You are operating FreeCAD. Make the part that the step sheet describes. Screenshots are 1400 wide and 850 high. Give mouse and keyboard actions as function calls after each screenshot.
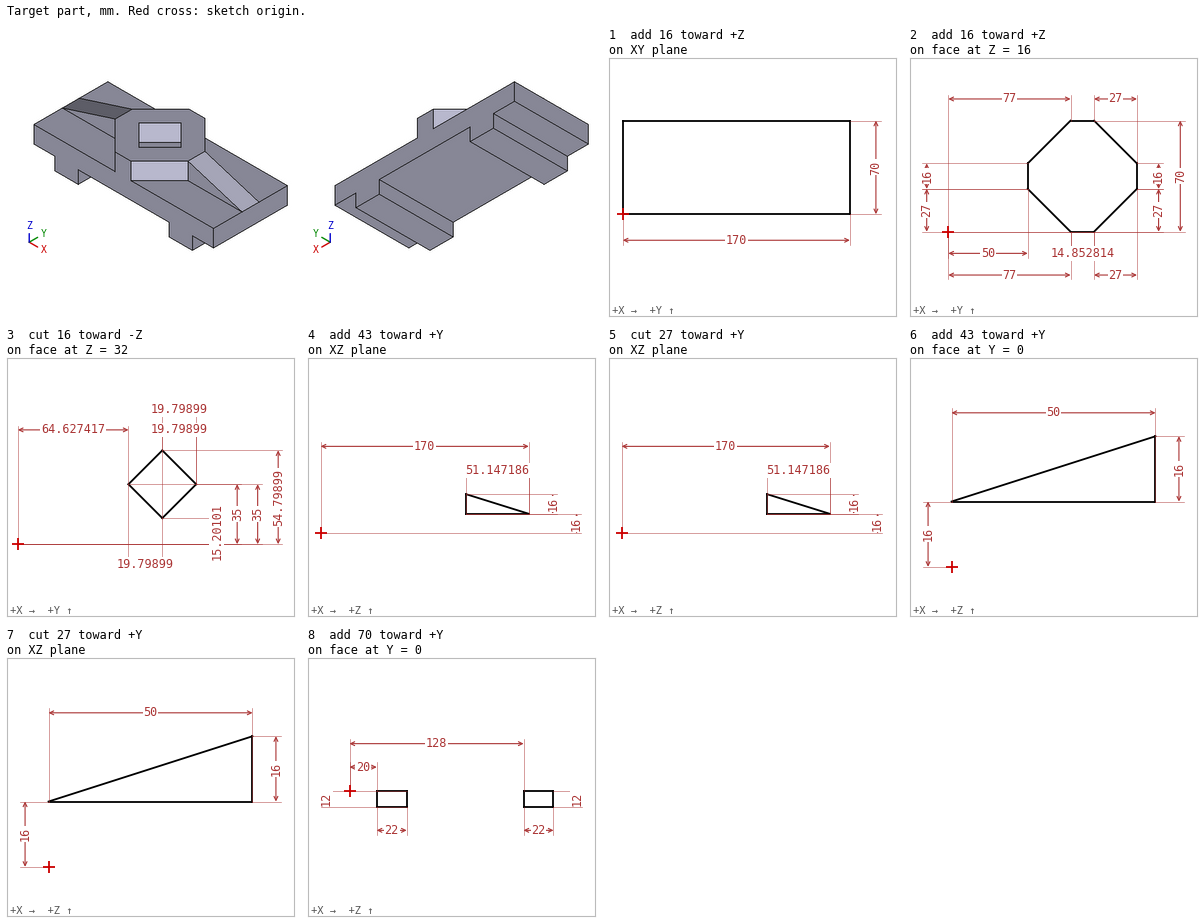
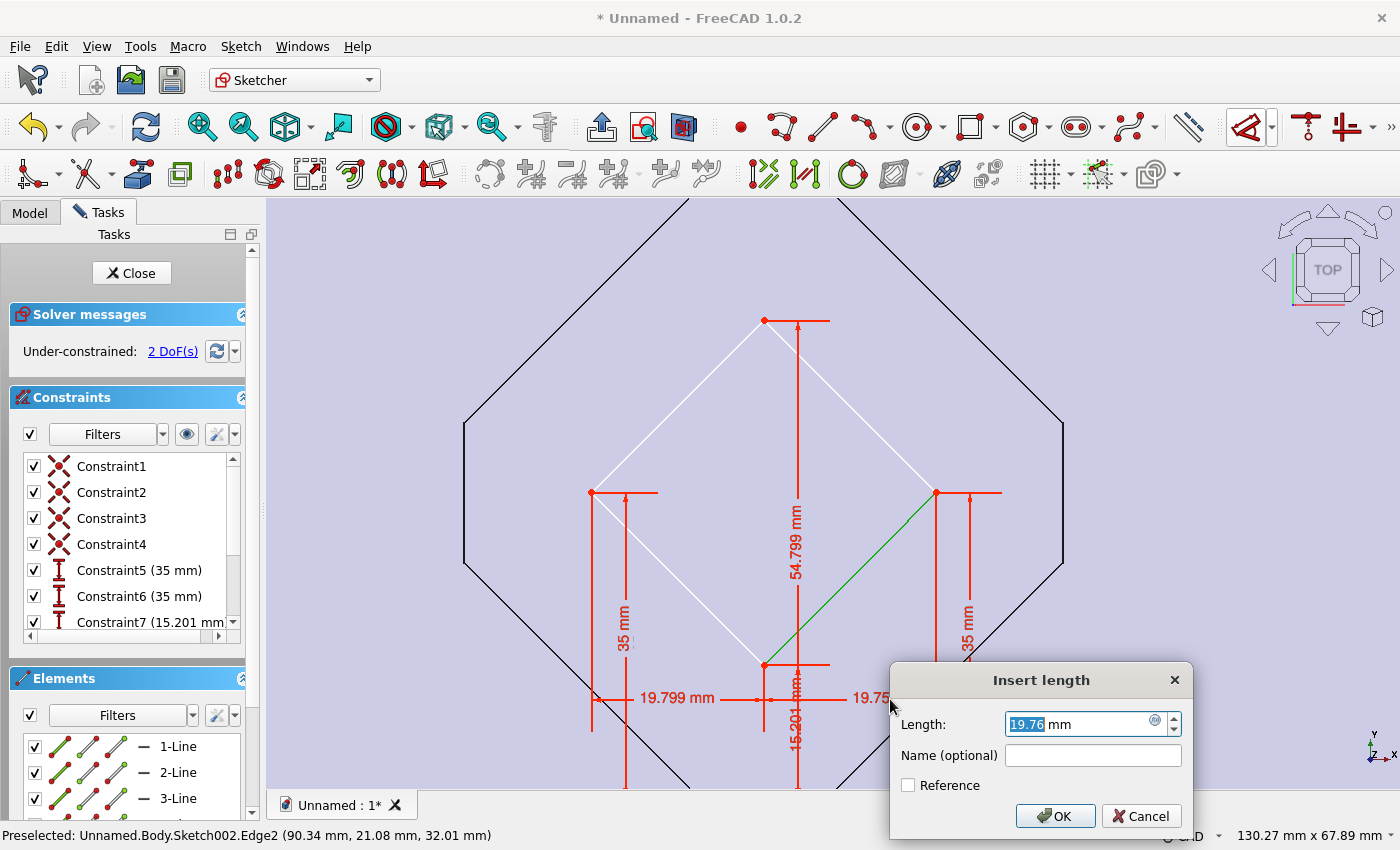
text(19.79899)
key(Return)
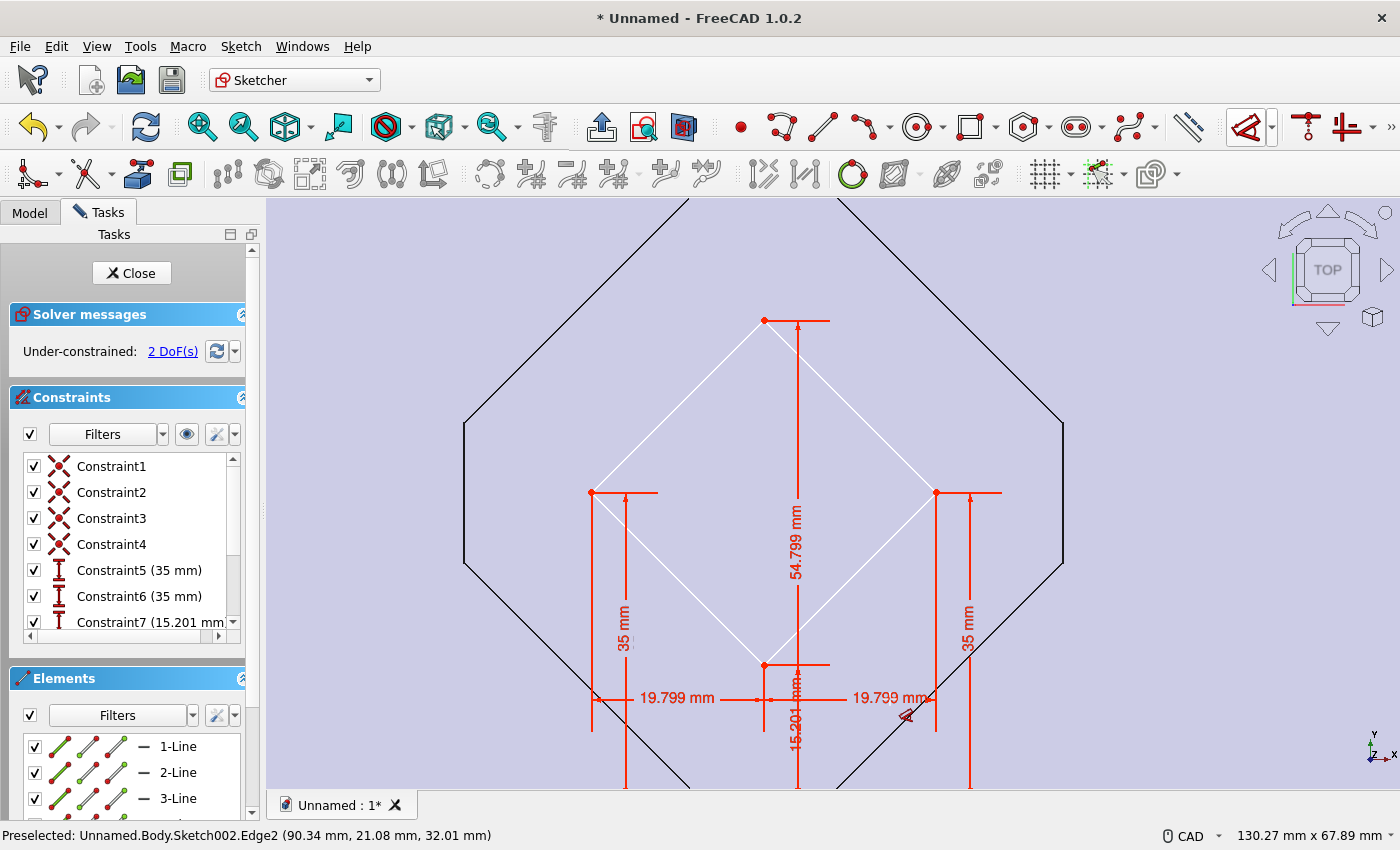
click(885, 441)
click(850, 287)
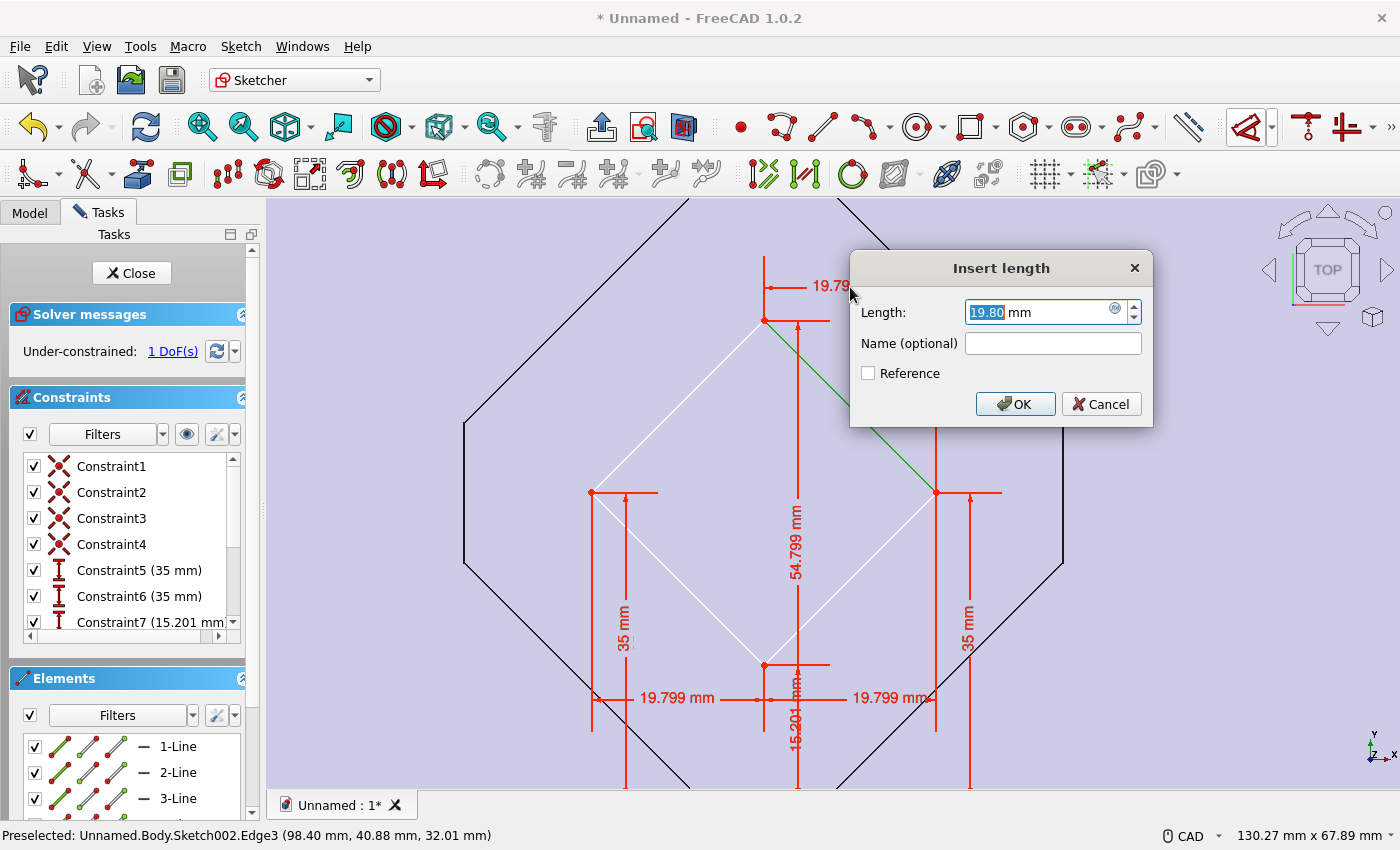
text(19.79899)
key(Return)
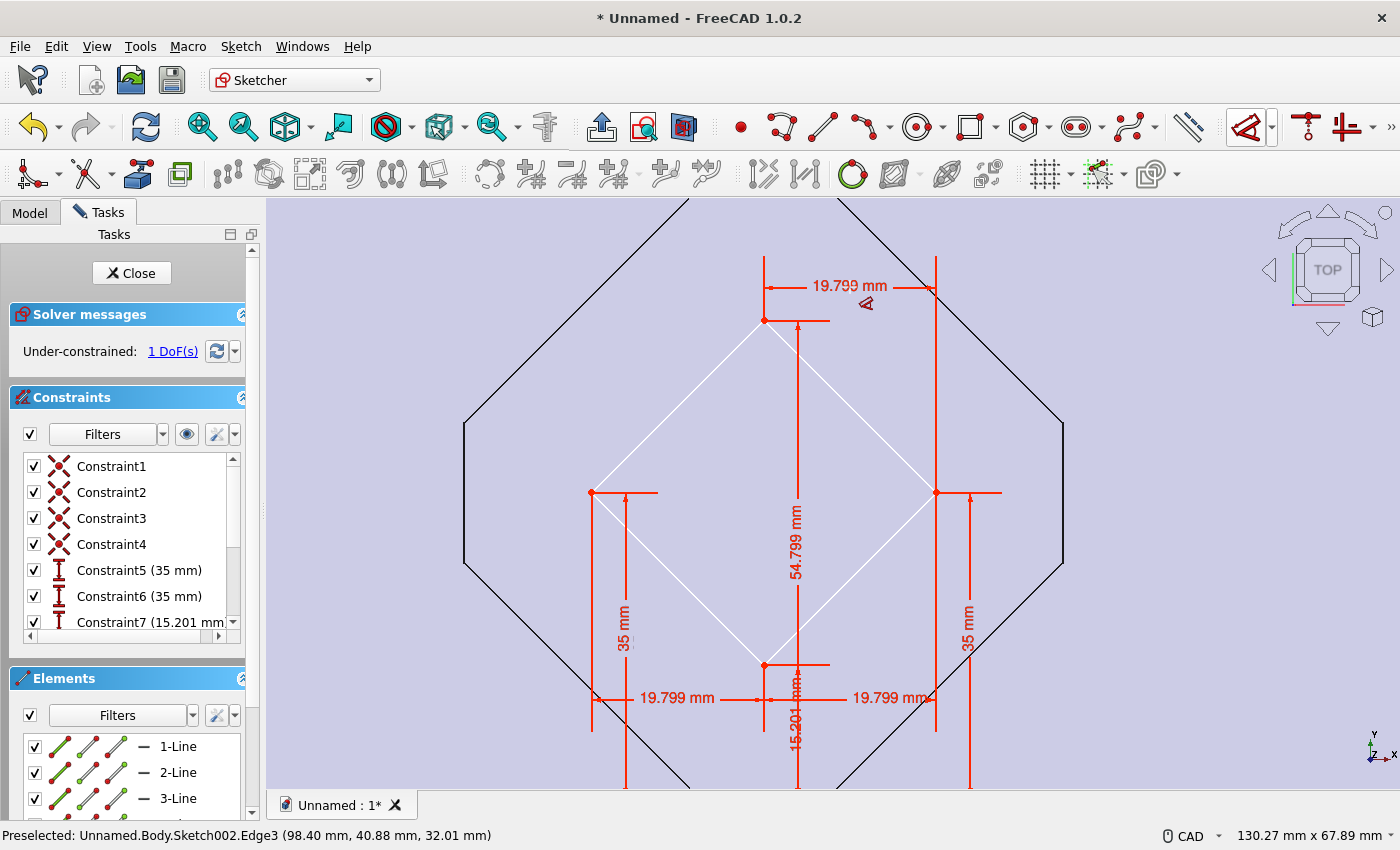
click(592, 493)
click(443, 459)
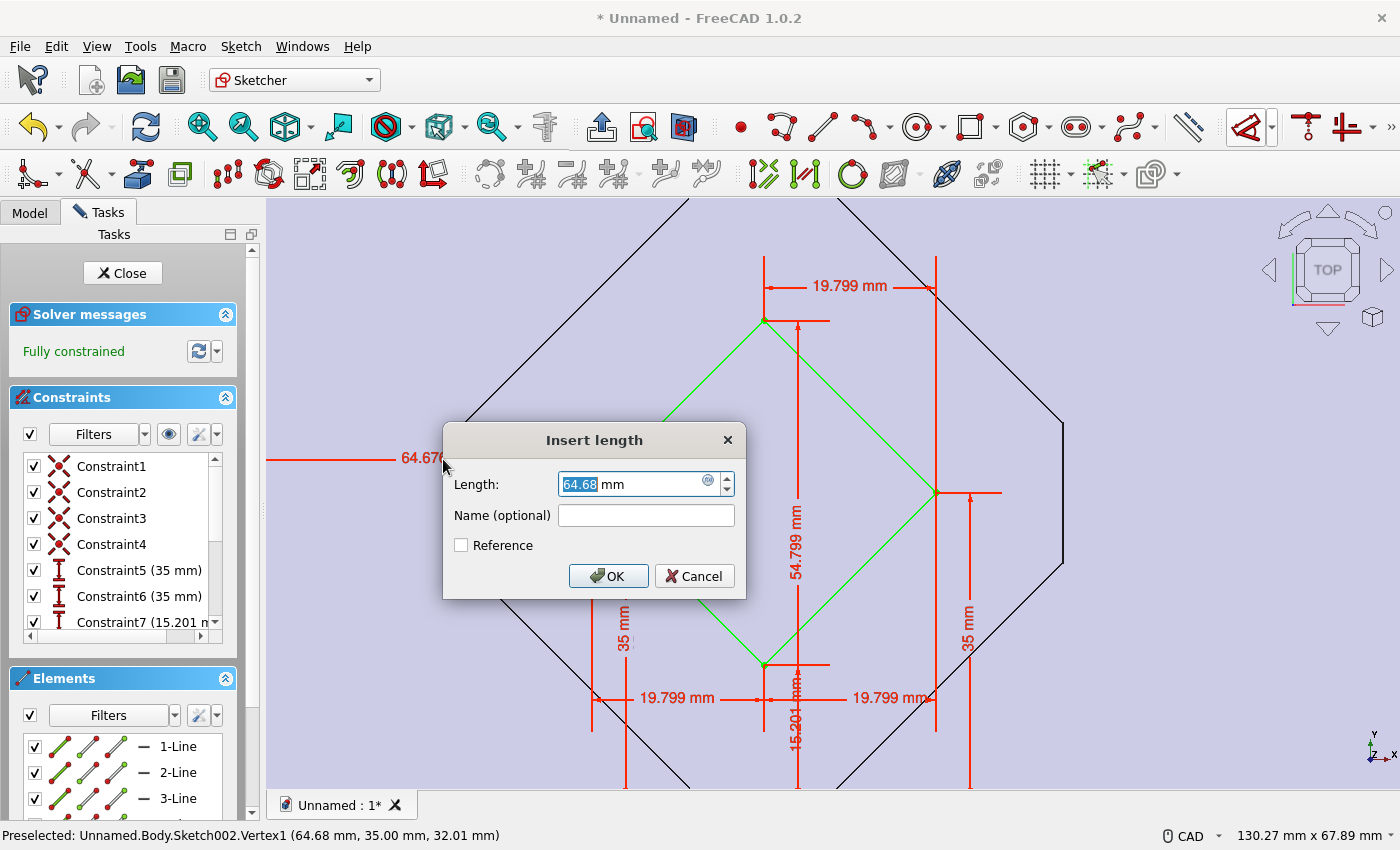
text(64.627417)
key(Return)
key(Escape)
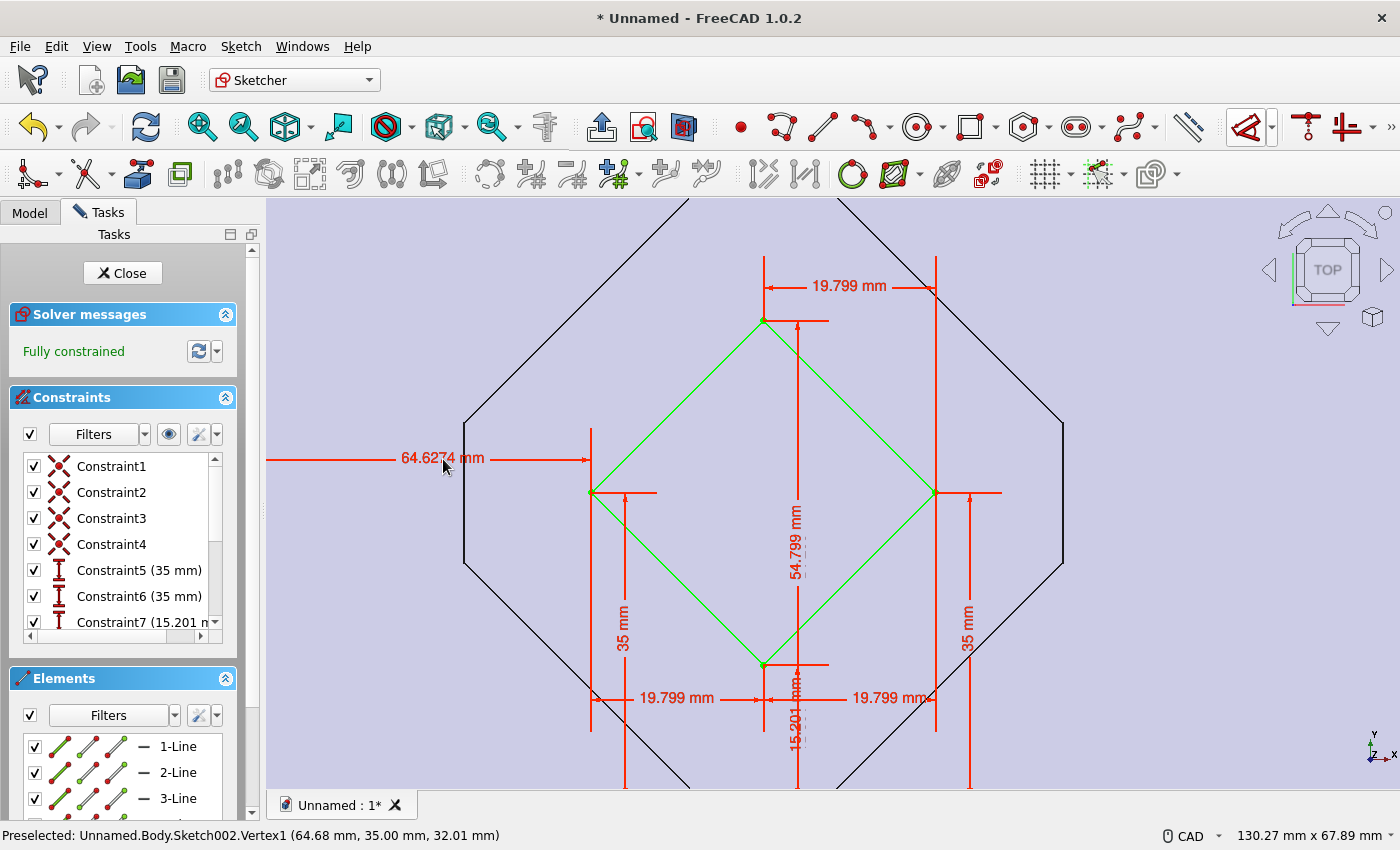
click(123, 273)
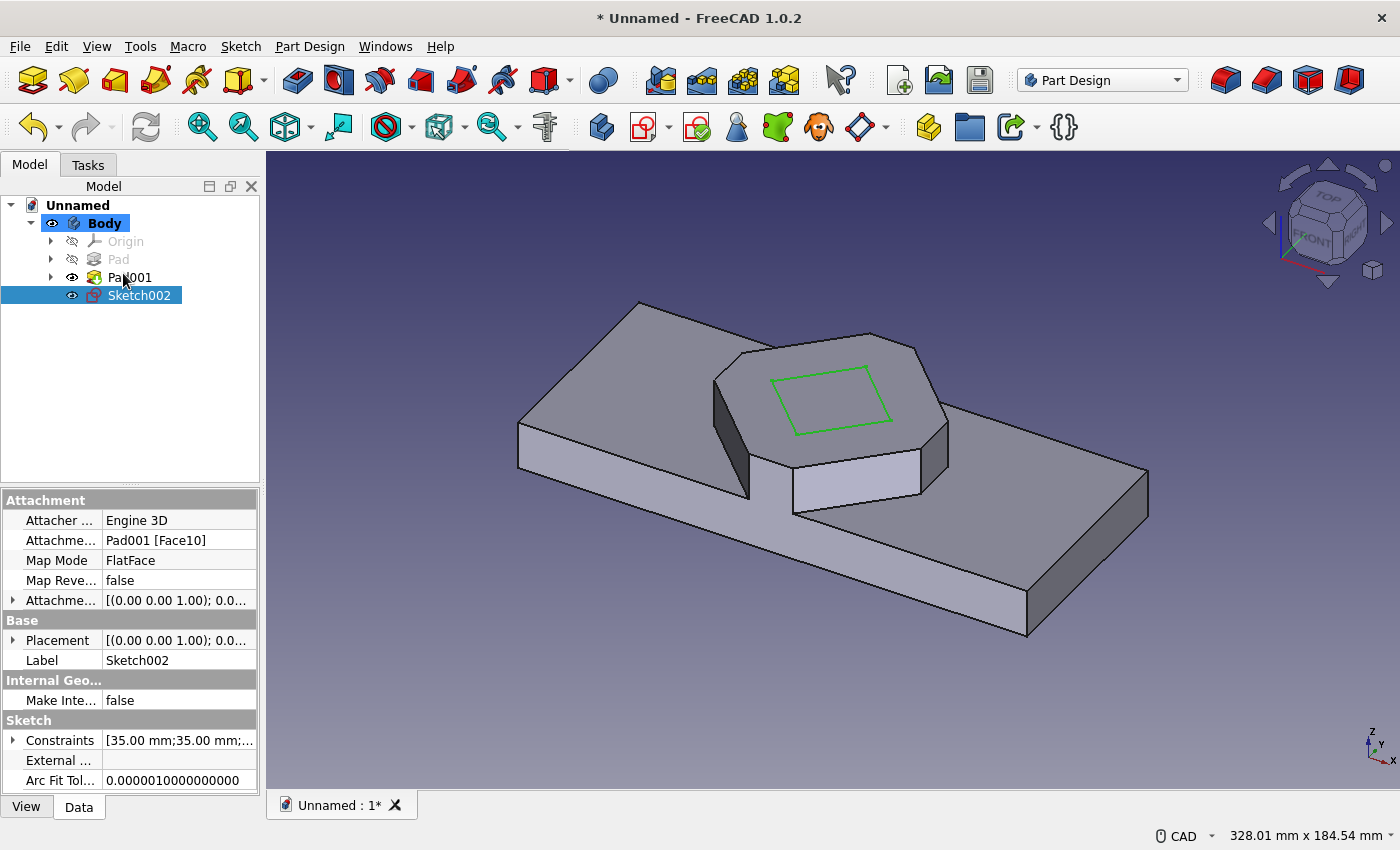
click(298, 80)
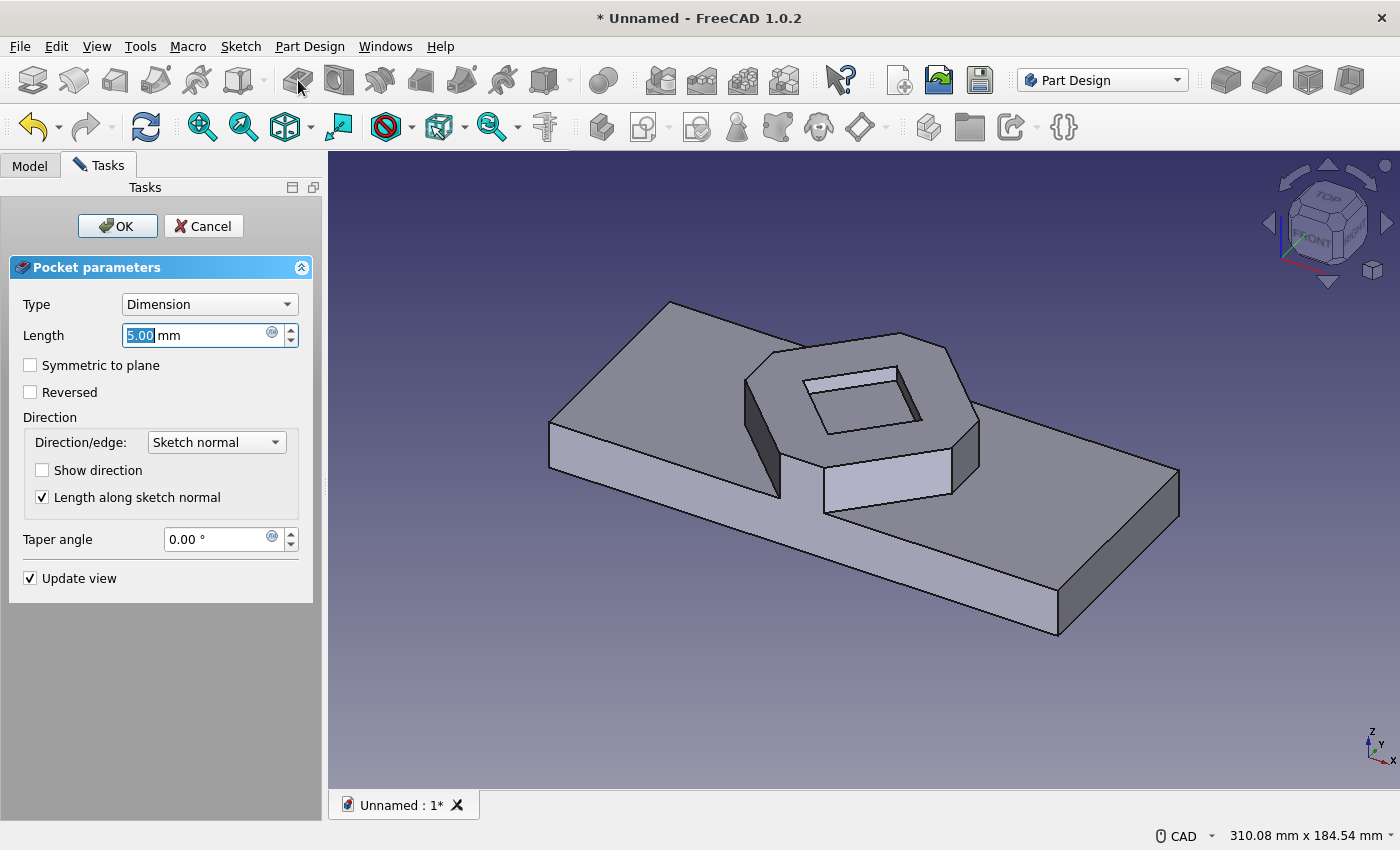
text(16)
key(Tab)